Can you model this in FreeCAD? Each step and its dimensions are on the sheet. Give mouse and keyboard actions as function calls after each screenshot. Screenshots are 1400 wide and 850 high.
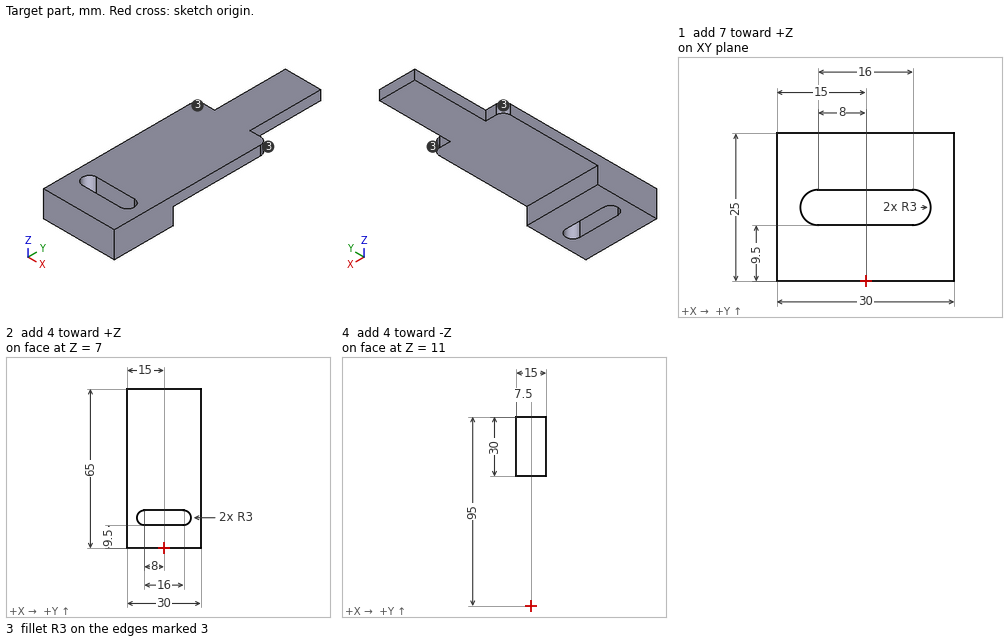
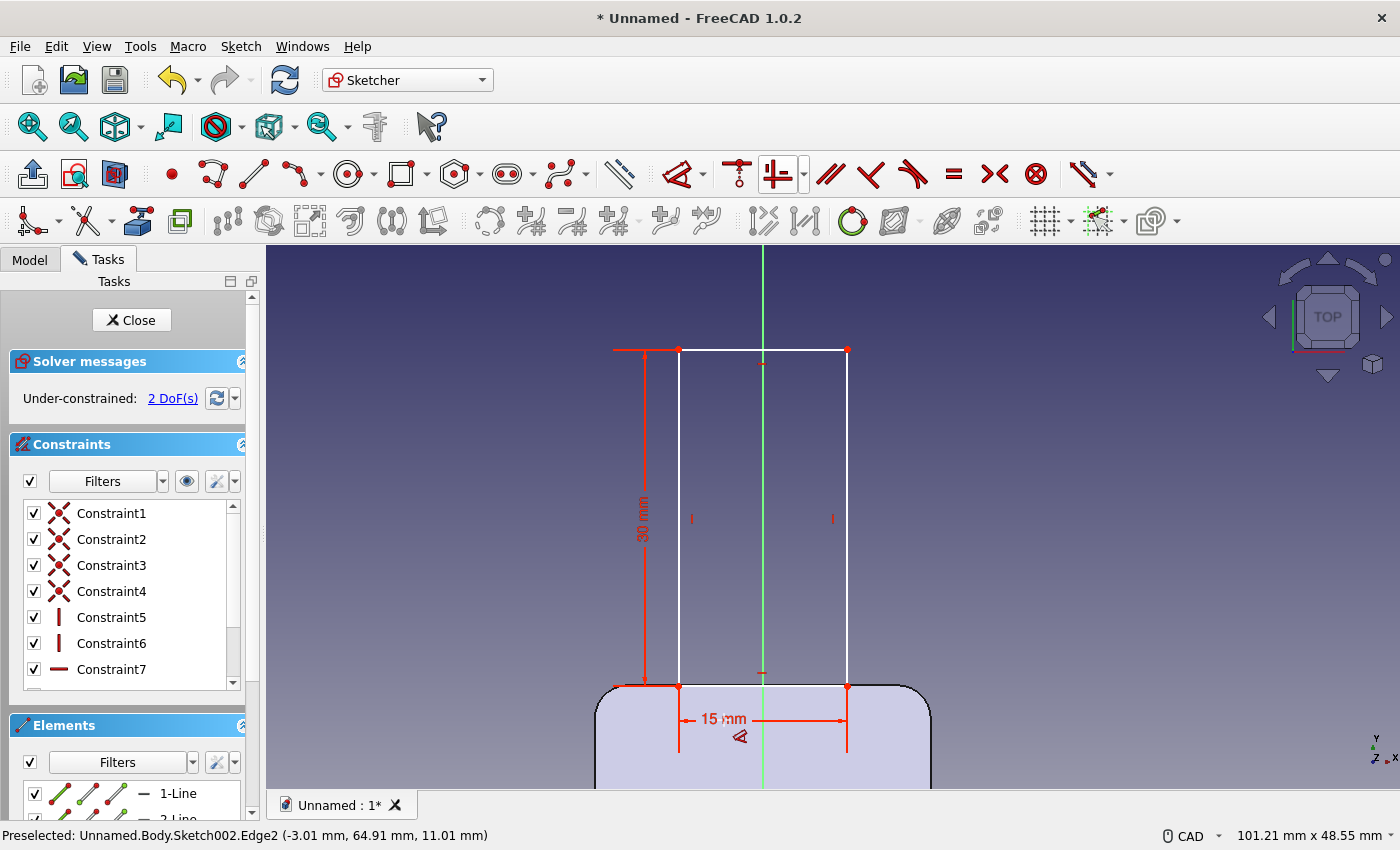
click(679, 350)
click(645, 555)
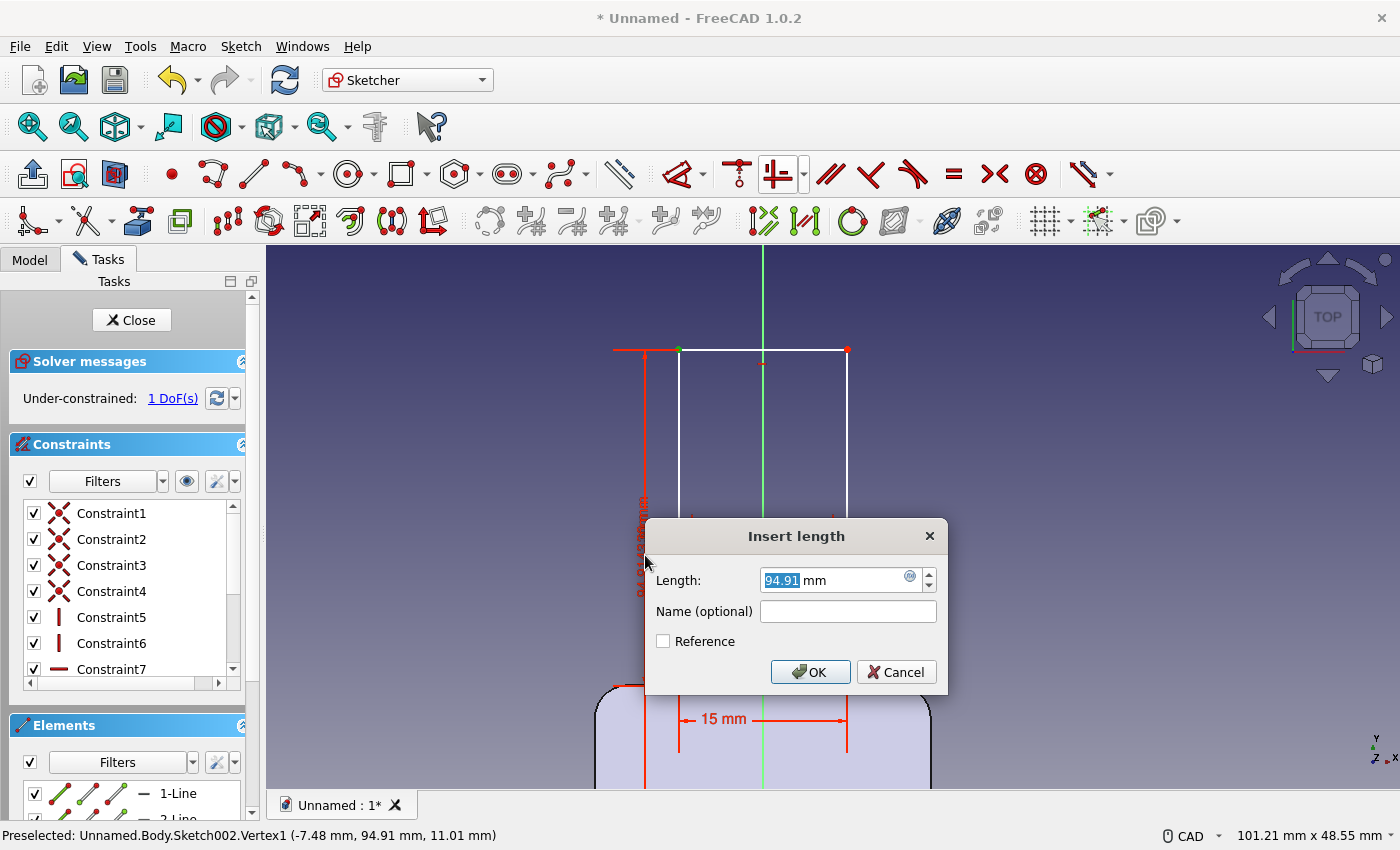
text(95)
key(Return)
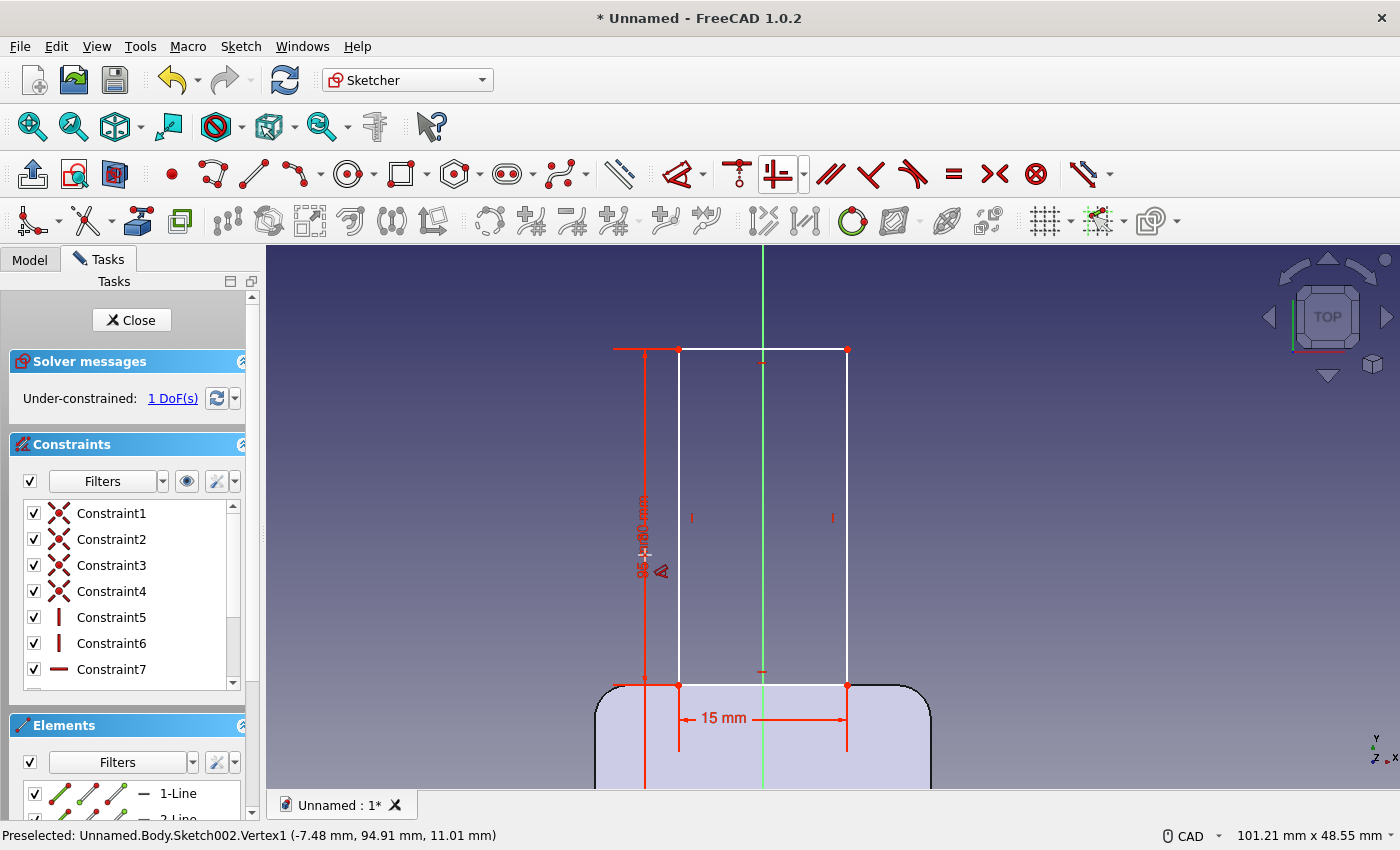
click(679, 349)
click(721, 315)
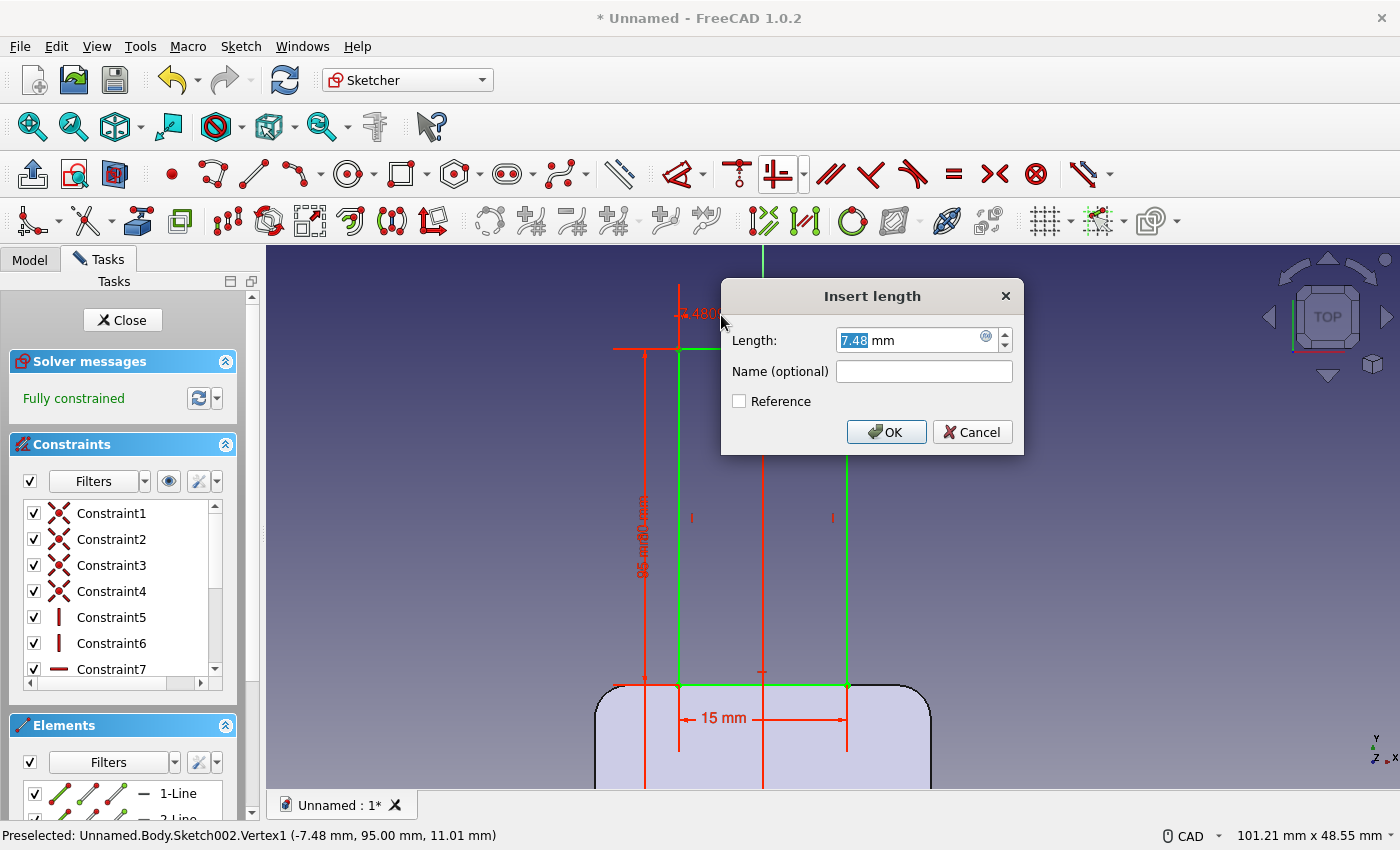
text(7.5)
key(Return)
key(Escape)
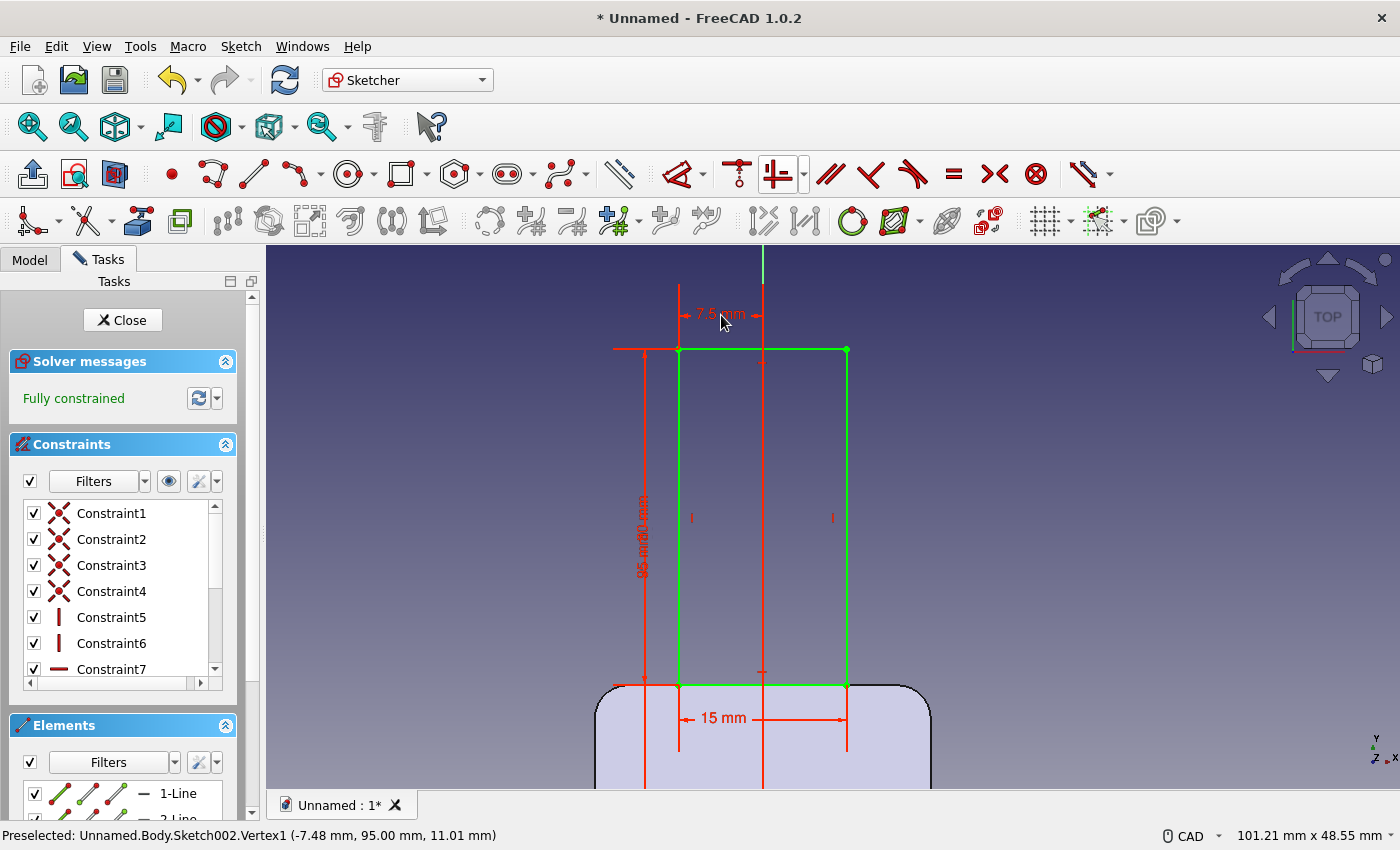
click(123, 320)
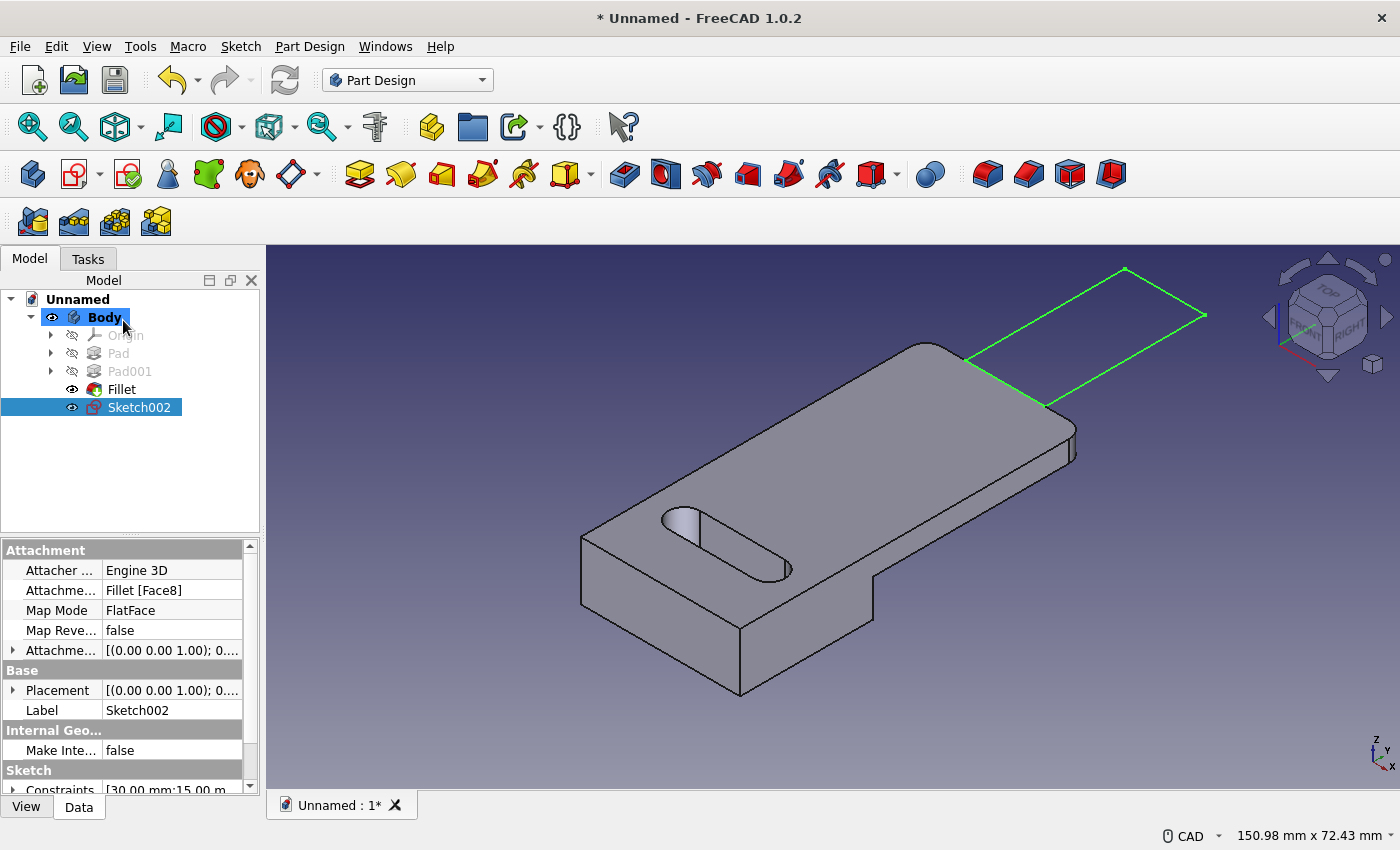
click(360, 174)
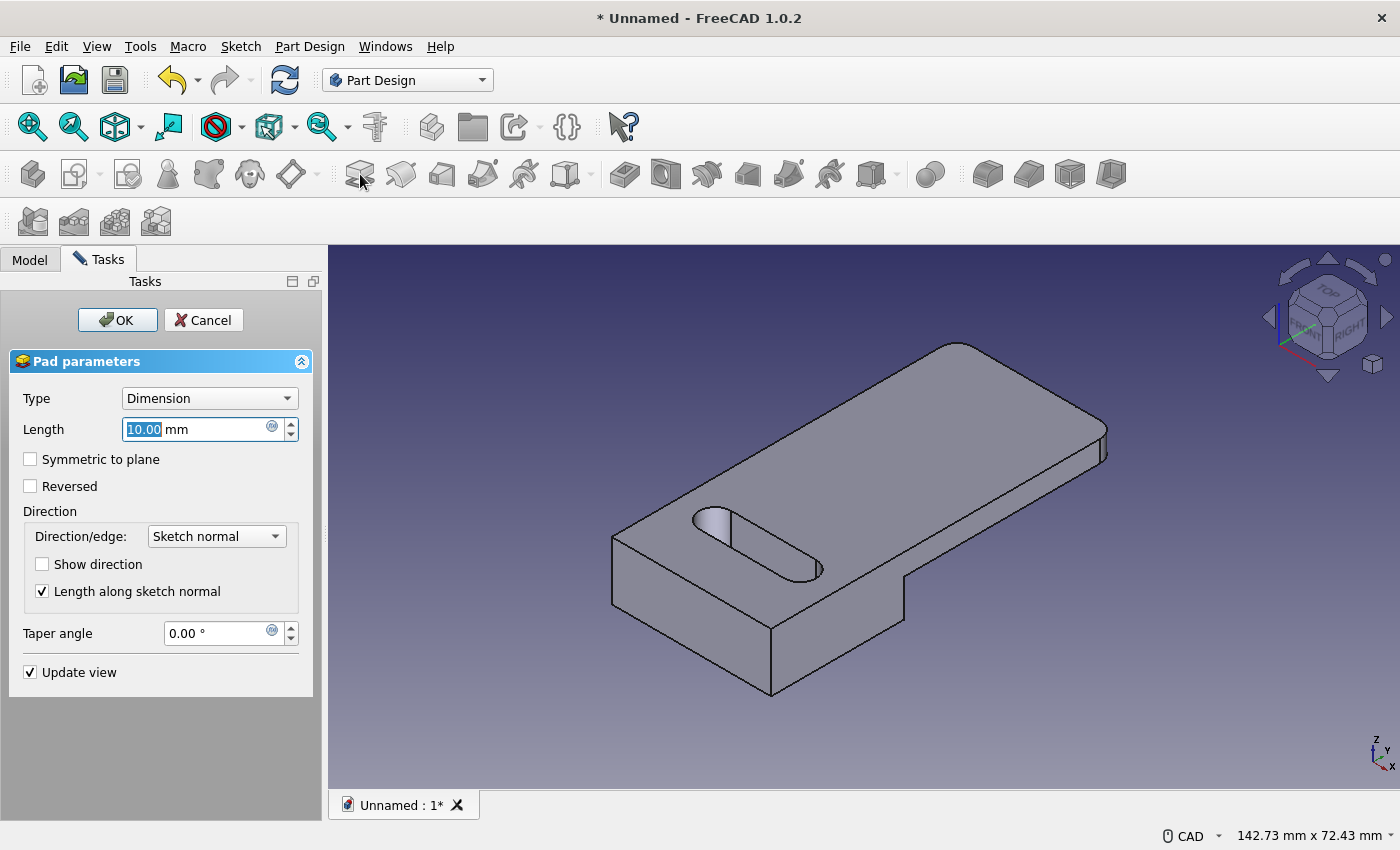
text(4)
key(Tab)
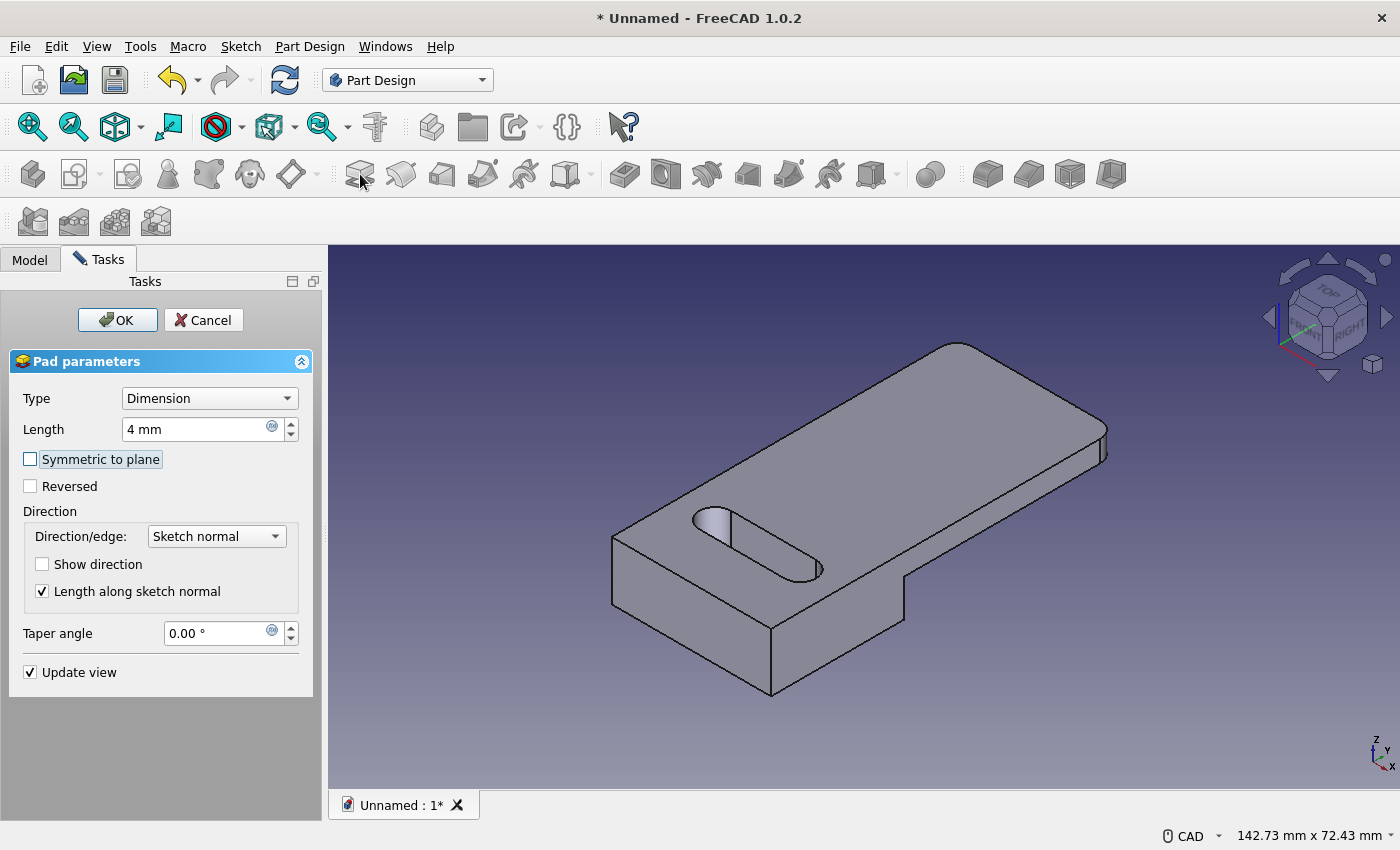
click(31, 486)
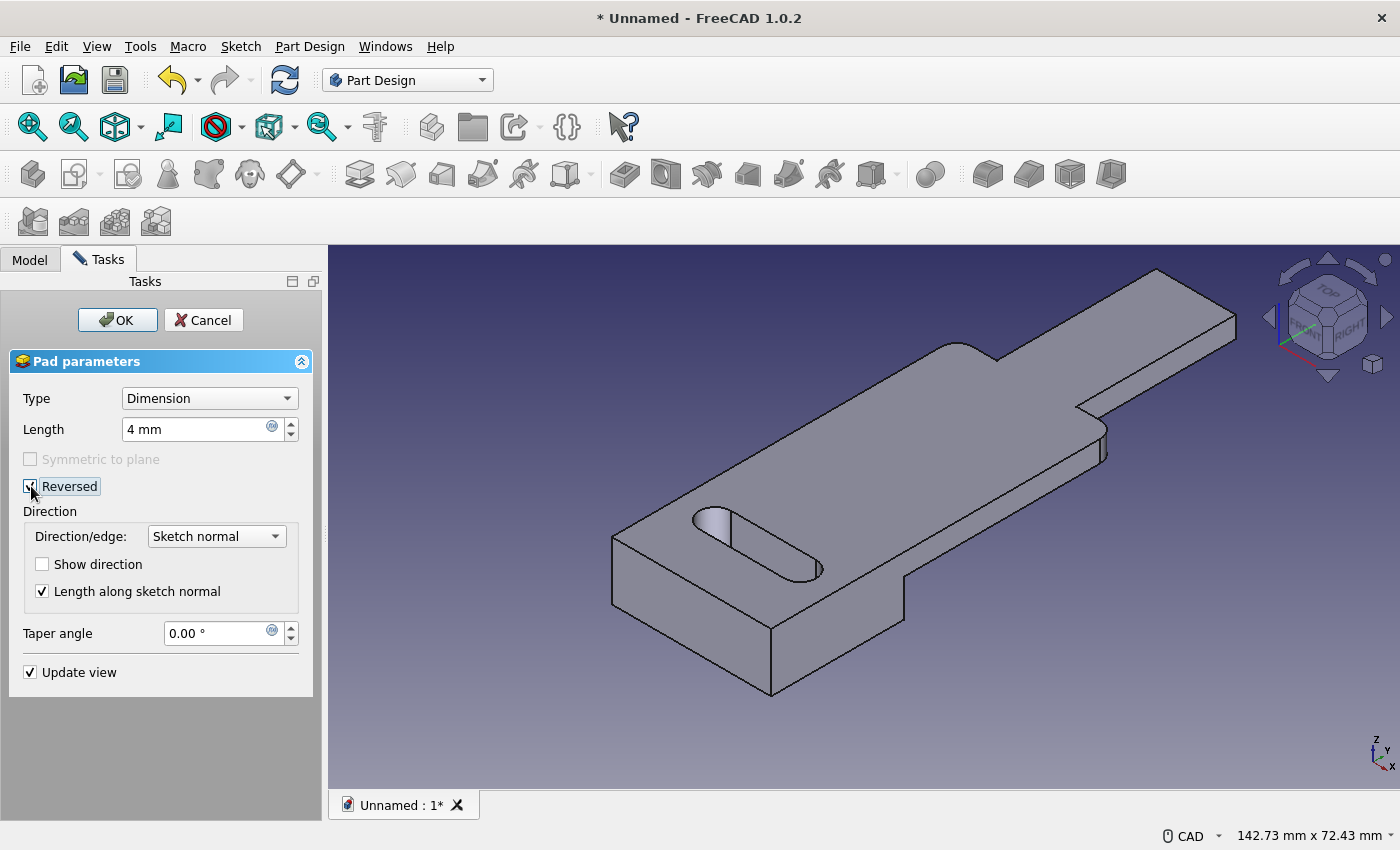
click(118, 320)